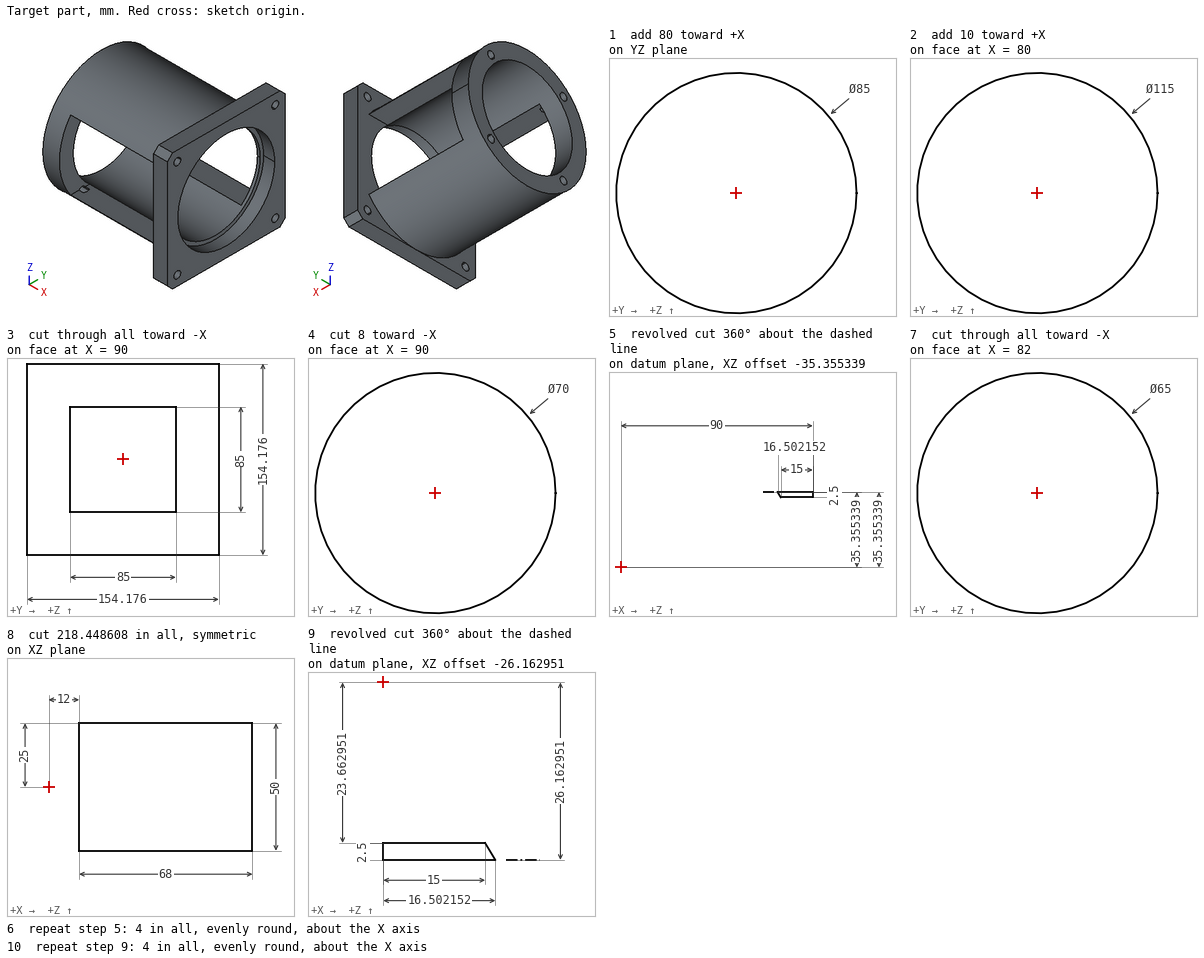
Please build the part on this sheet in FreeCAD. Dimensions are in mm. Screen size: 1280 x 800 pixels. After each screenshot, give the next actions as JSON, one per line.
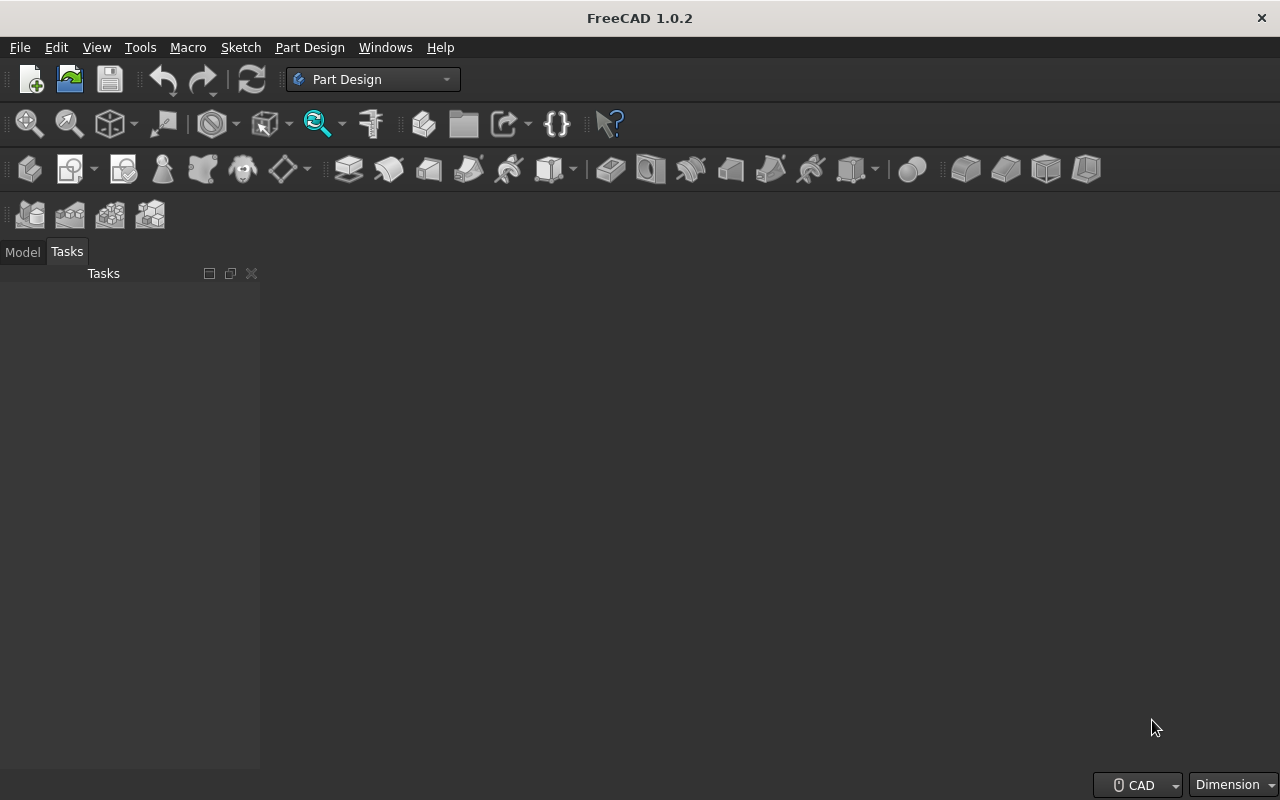
{"action": "left_click", "coordinate": [30, 80]}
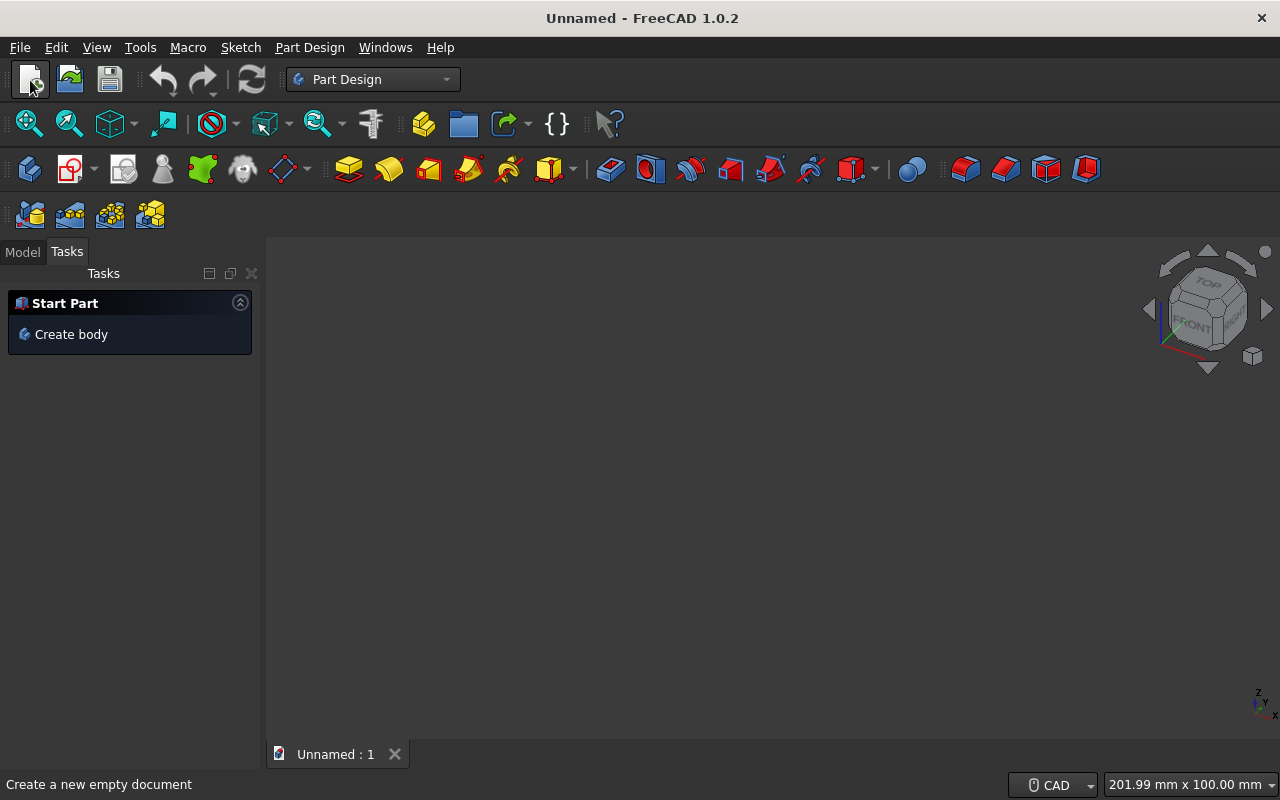
{"action": "left_click", "coordinate": [70, 170]}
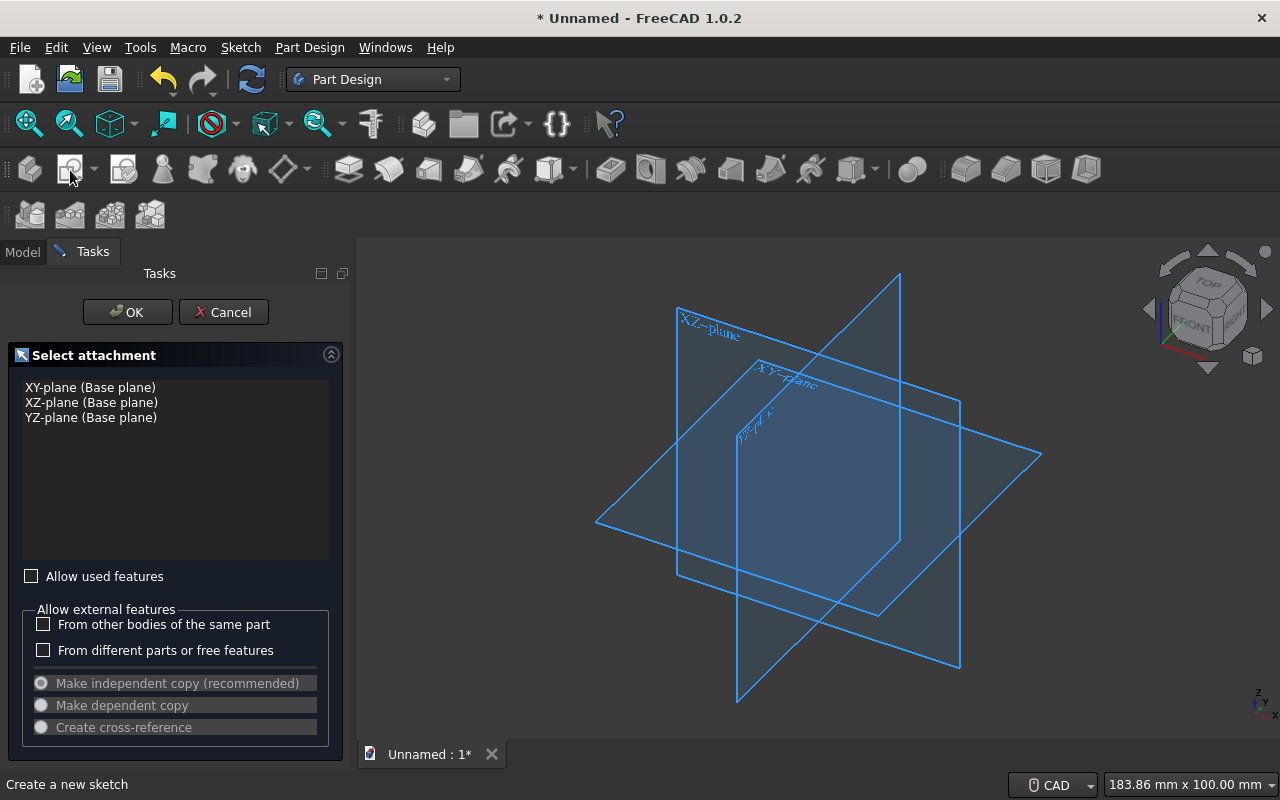
{"action": "left_click", "coordinate": [82, 418]}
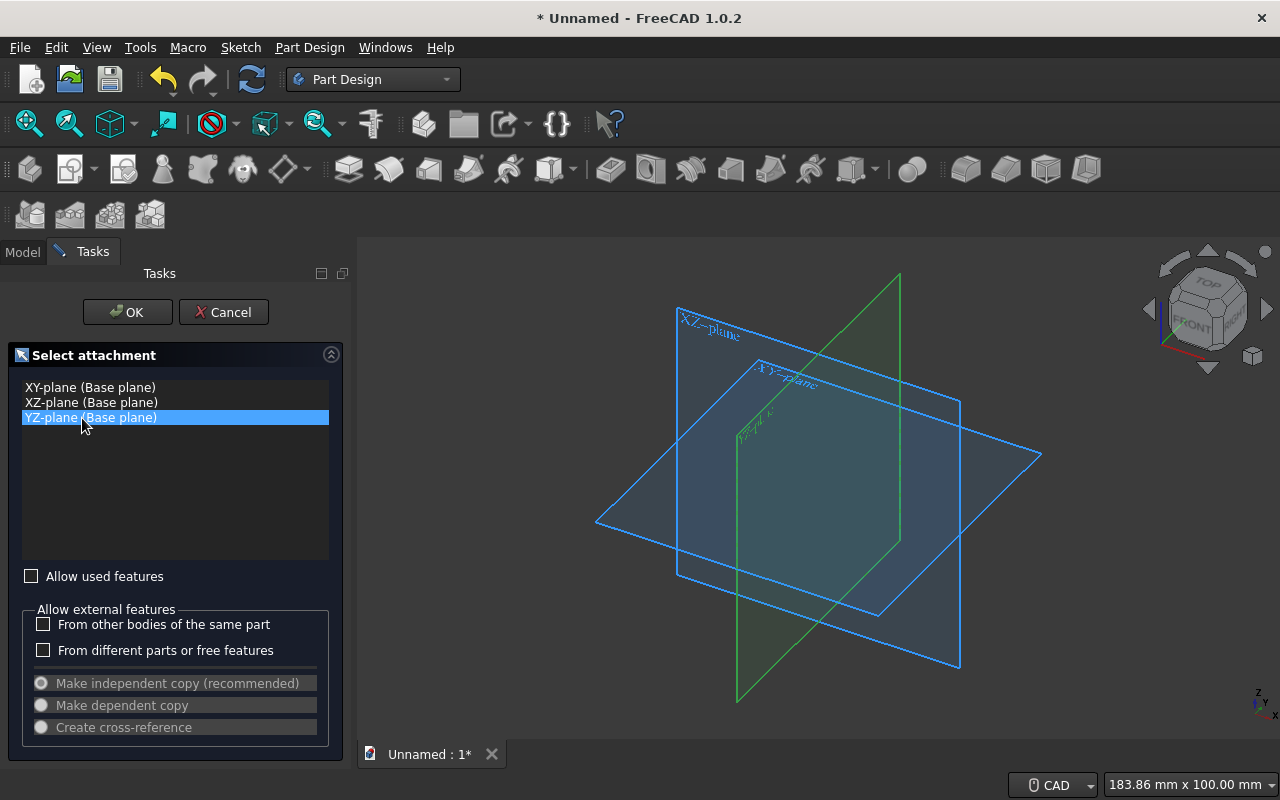
{"action": "left_click", "coordinate": [128, 312]}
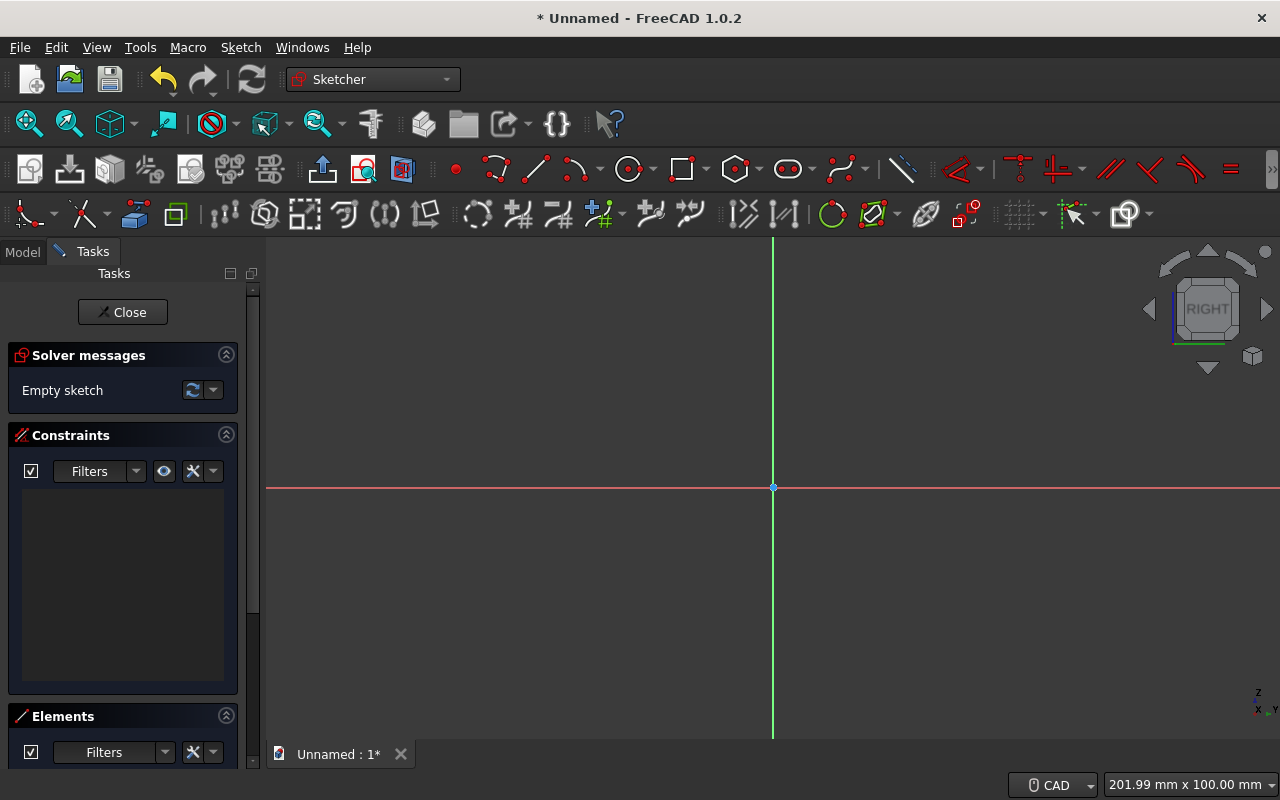
{"action": "scroll", "coordinate": [565, 488], "scroll_direction": "down", "scroll_amount": 2}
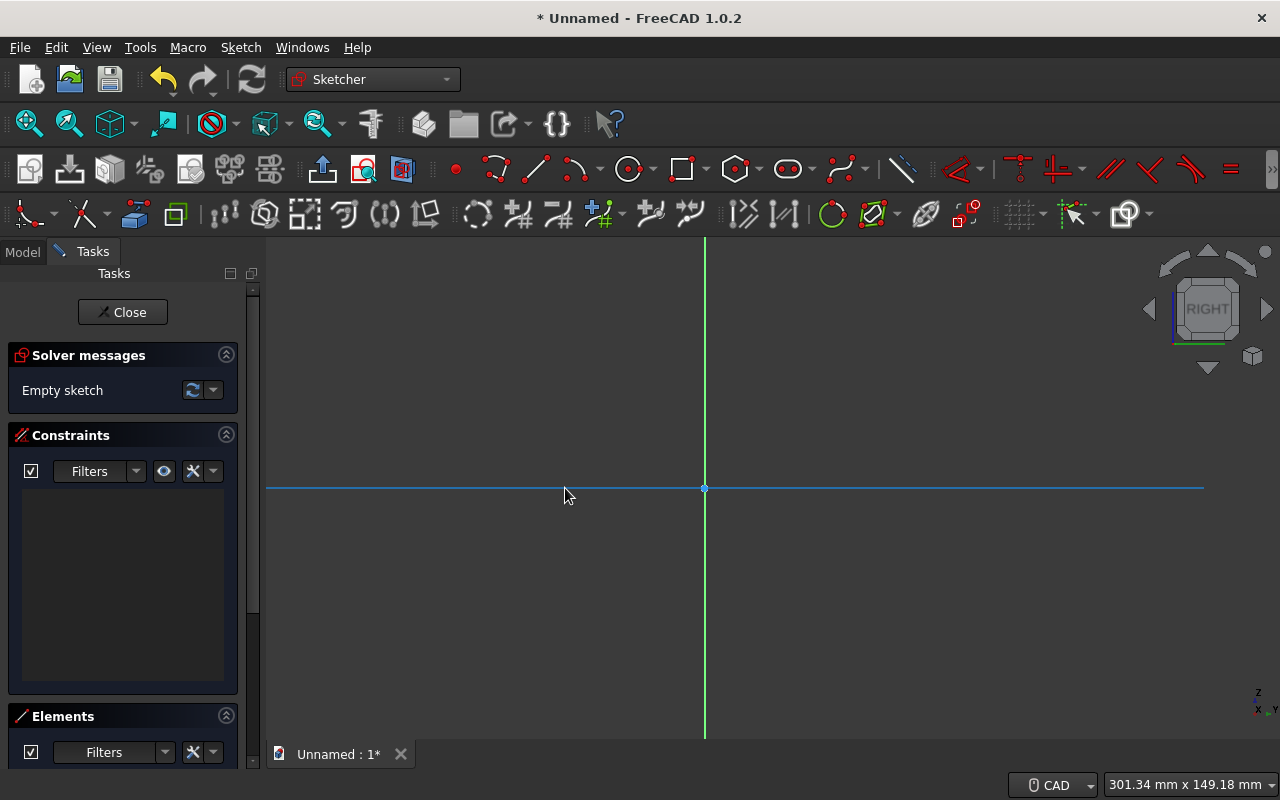
{"action": "key", "text": "g c"}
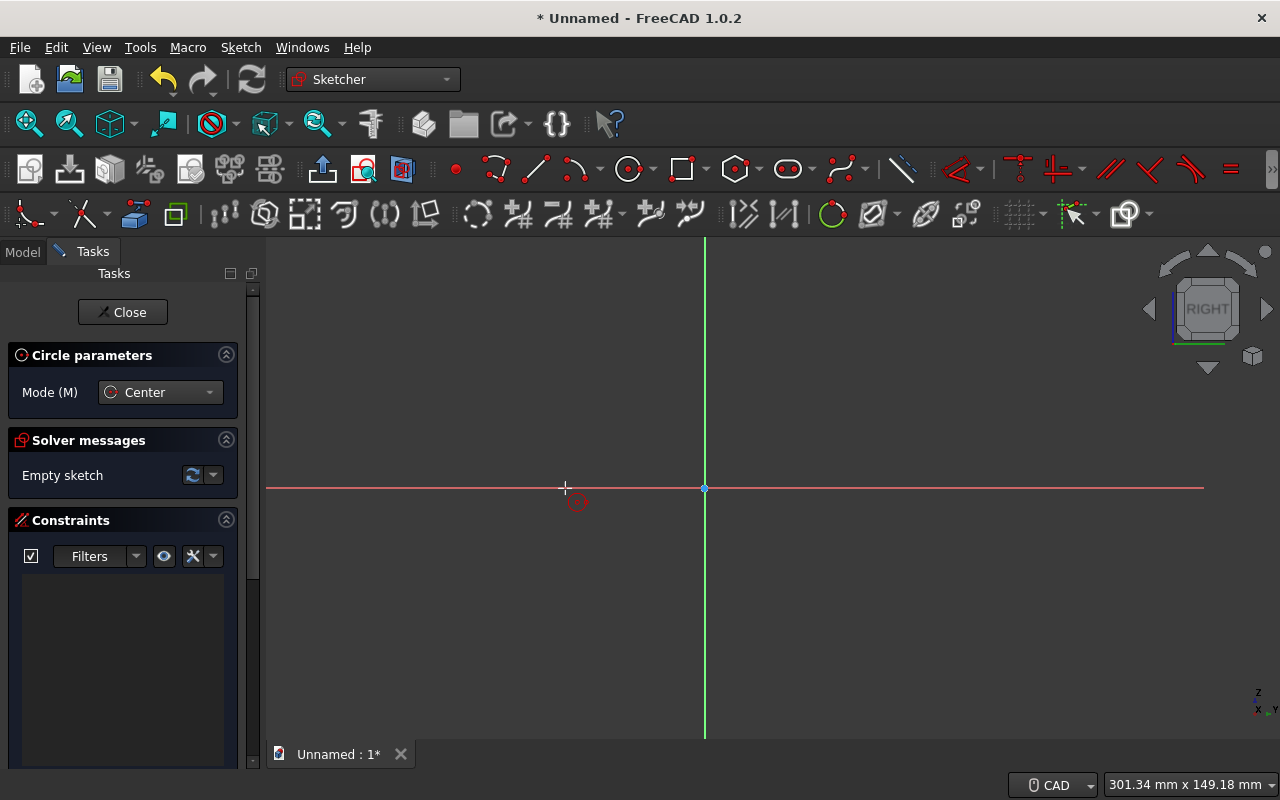
{"action": "left_click", "coordinate": [705, 488]}
{"action": "mouse_move", "coordinate": [806, 387]}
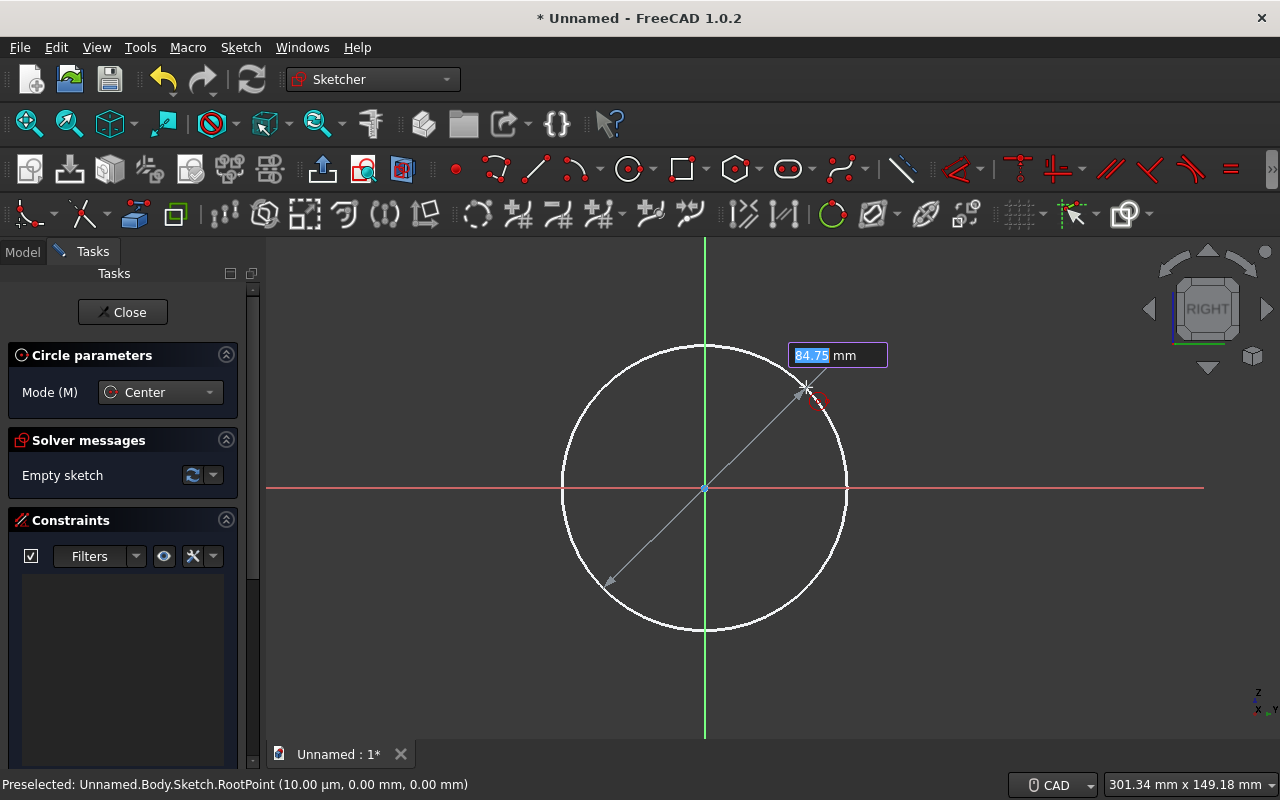
{"action": "type", "text": "85"}
{"action": "key", "text": "Return"}
{"action": "key", "text": "Escape"}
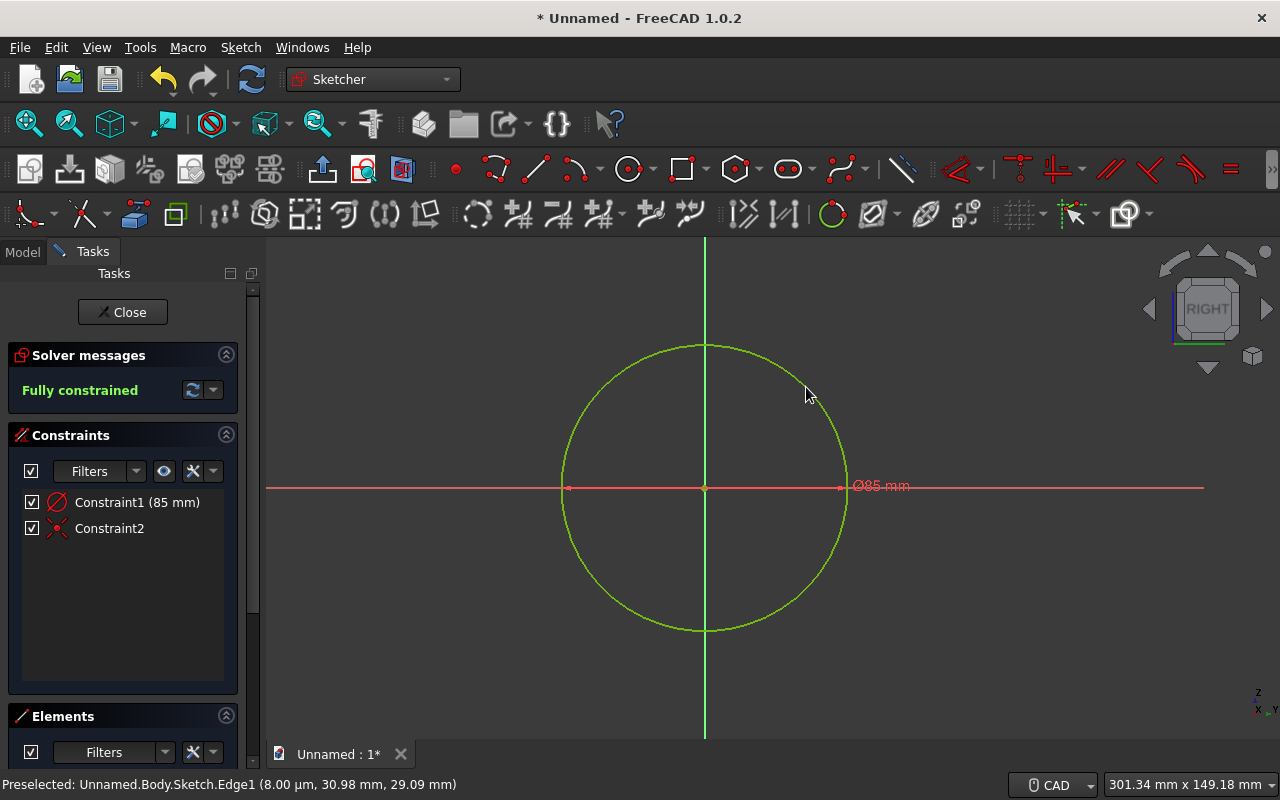
{"action": "left_click", "coordinate": [123, 312]}